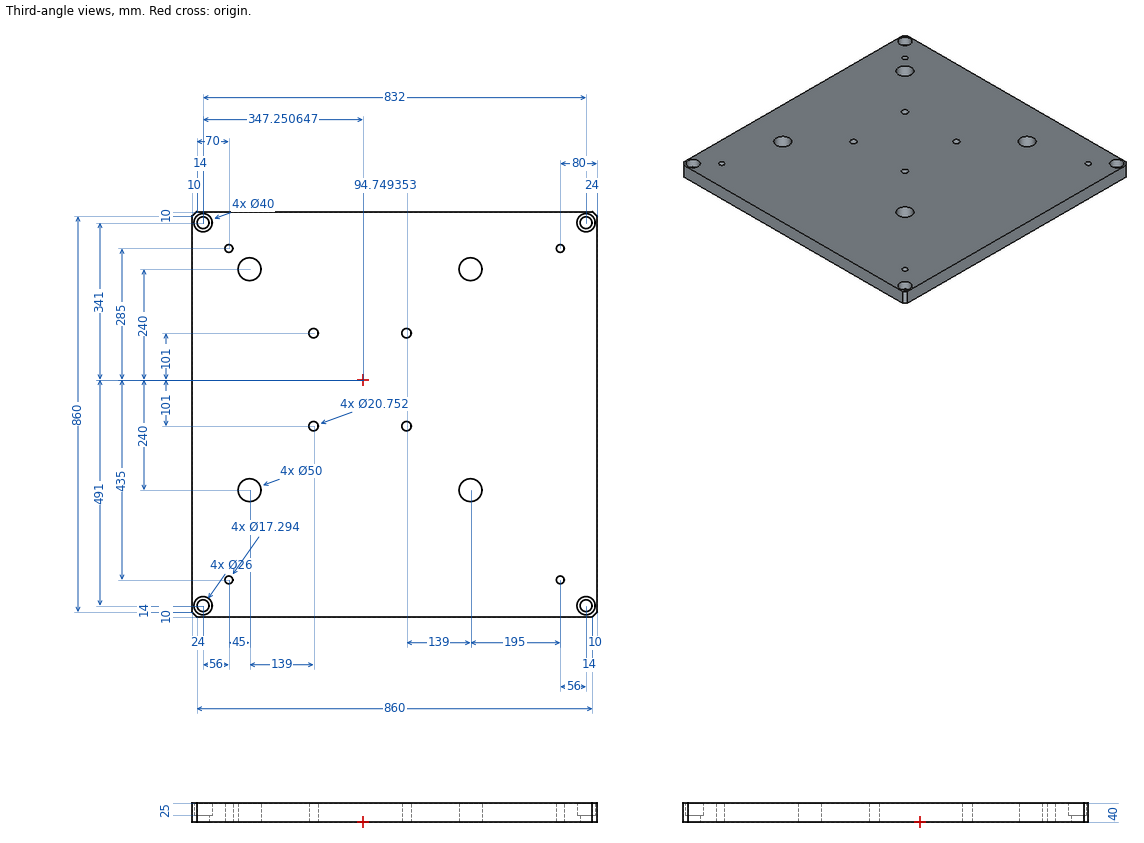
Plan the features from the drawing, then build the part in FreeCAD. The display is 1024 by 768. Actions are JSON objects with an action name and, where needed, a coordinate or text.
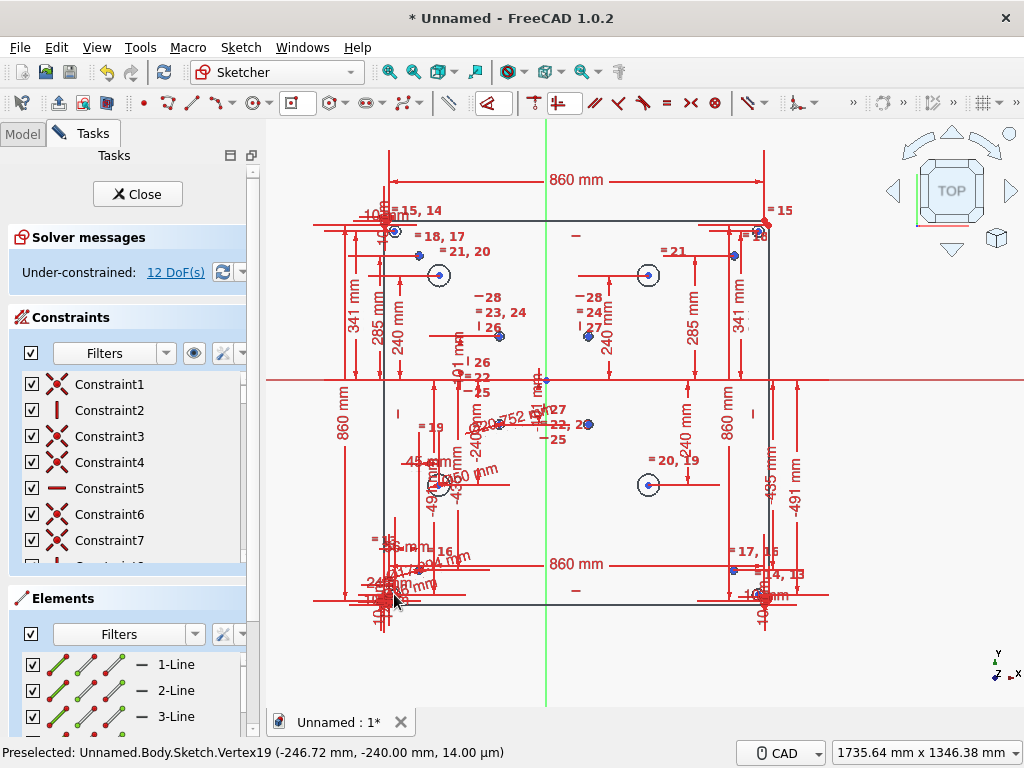
{"action": "scroll", "coordinate": [764, 605], "scroll_direction": "up", "scroll_amount": 10}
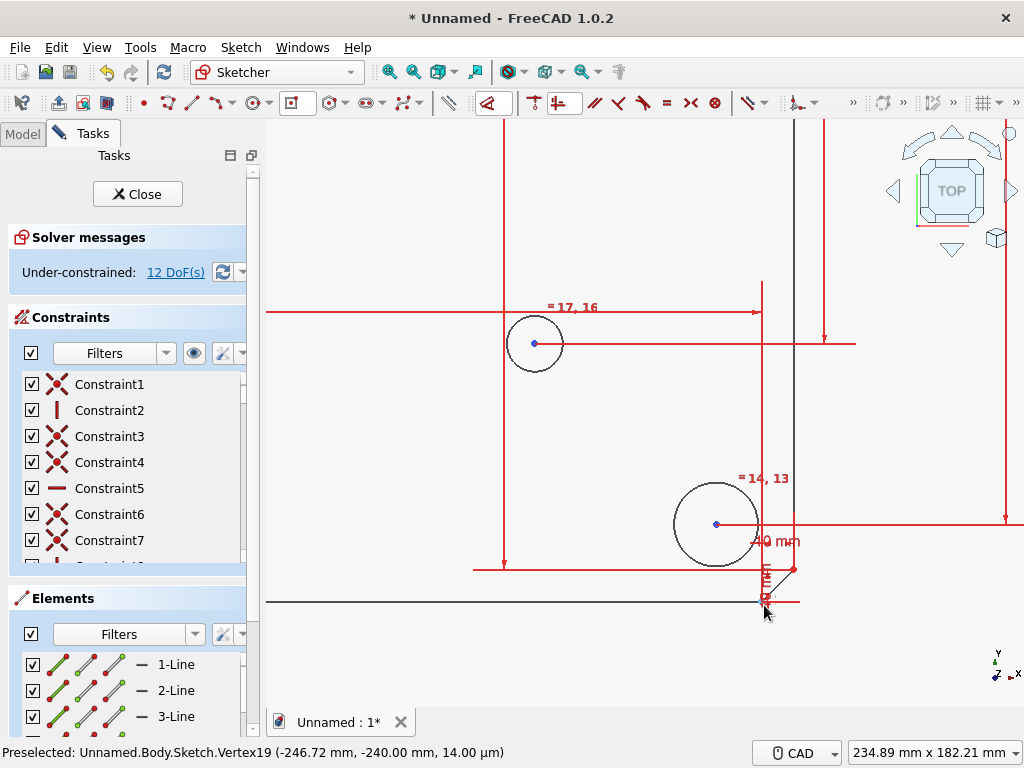
{"action": "left_click", "coordinate": [762, 602]}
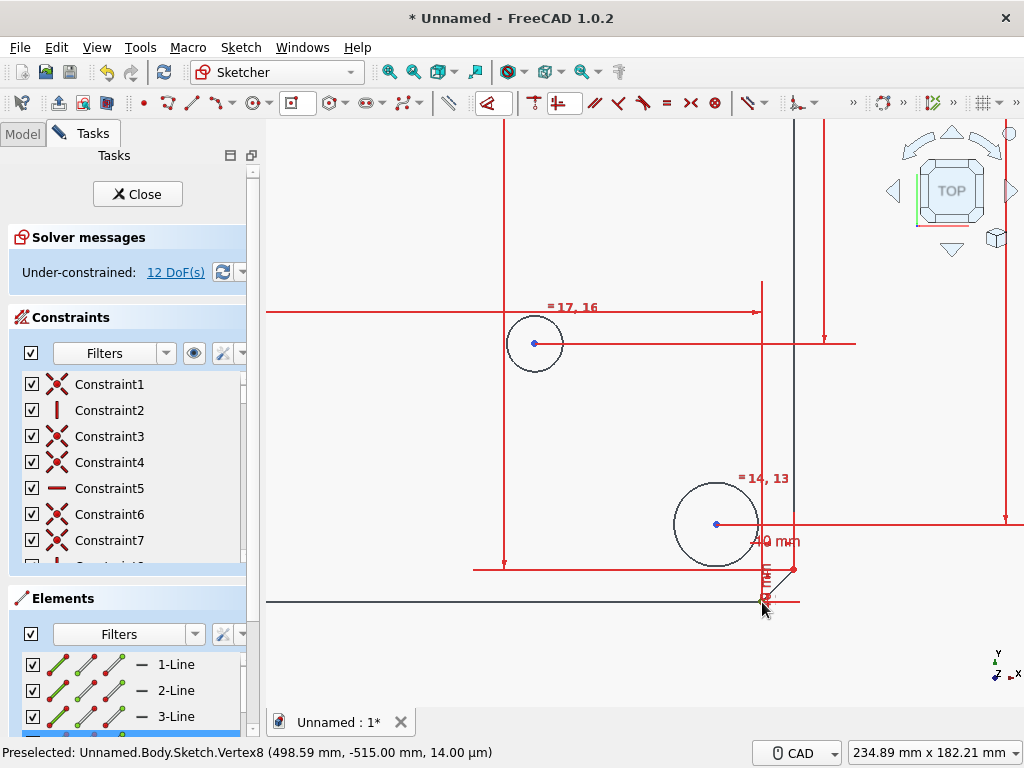
{"action": "left_click", "coordinate": [716, 525]}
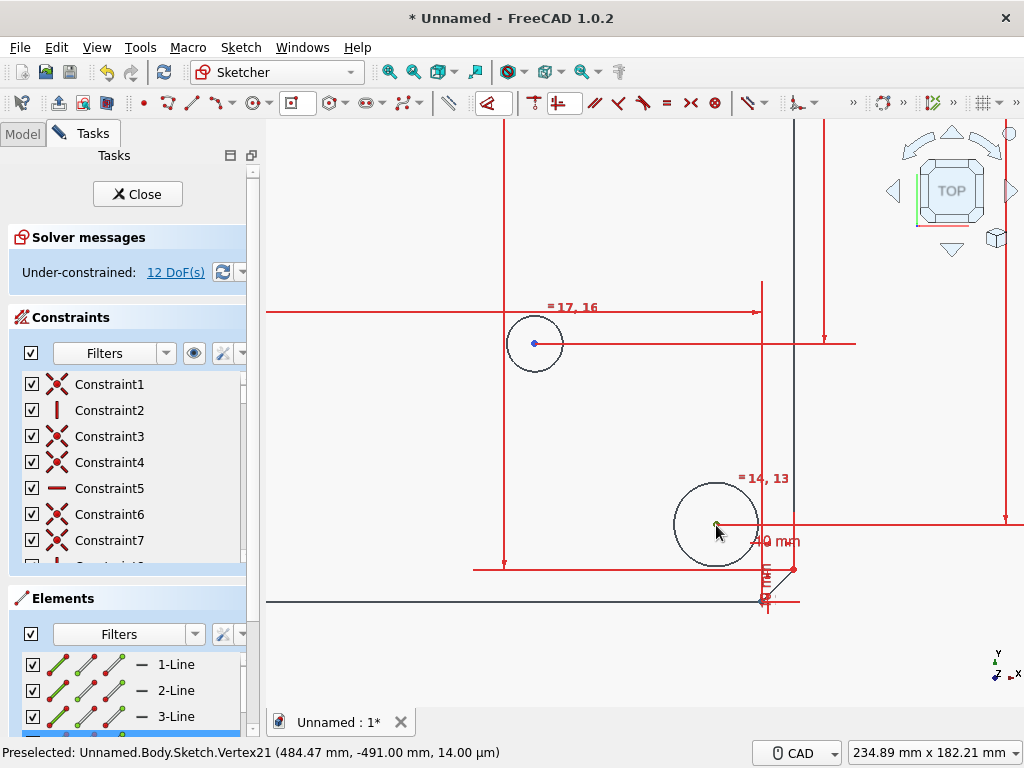
{"action": "key", "text": "l"}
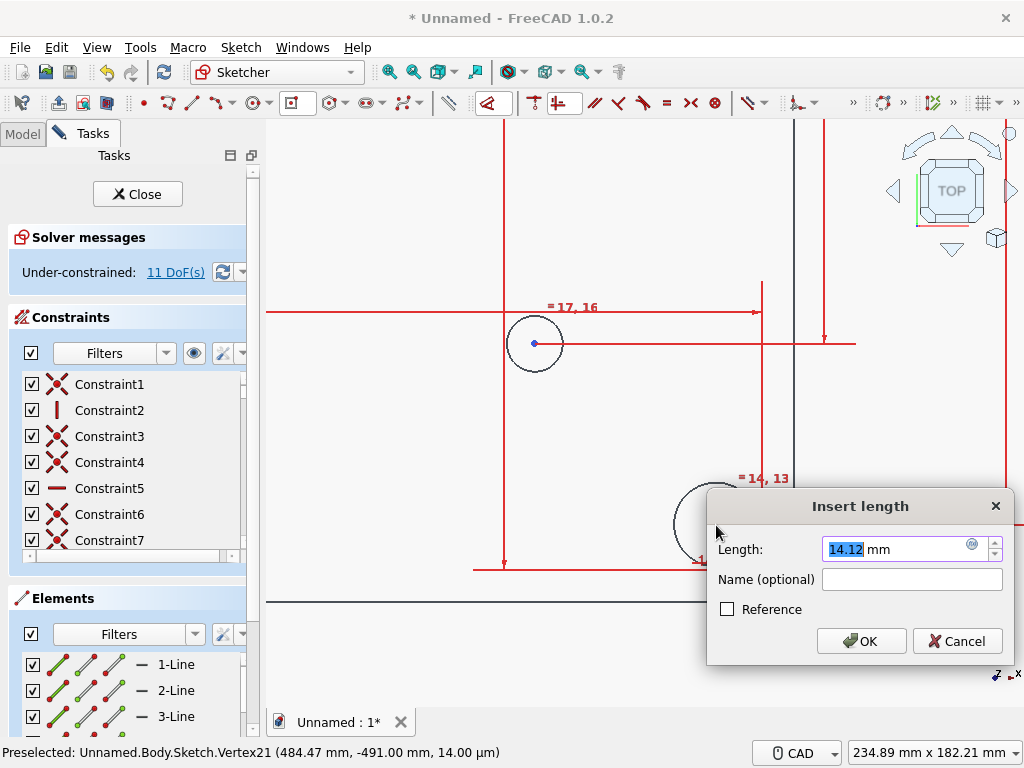
{"action": "type", "text": "14"}
{"action": "key", "text": "Return"}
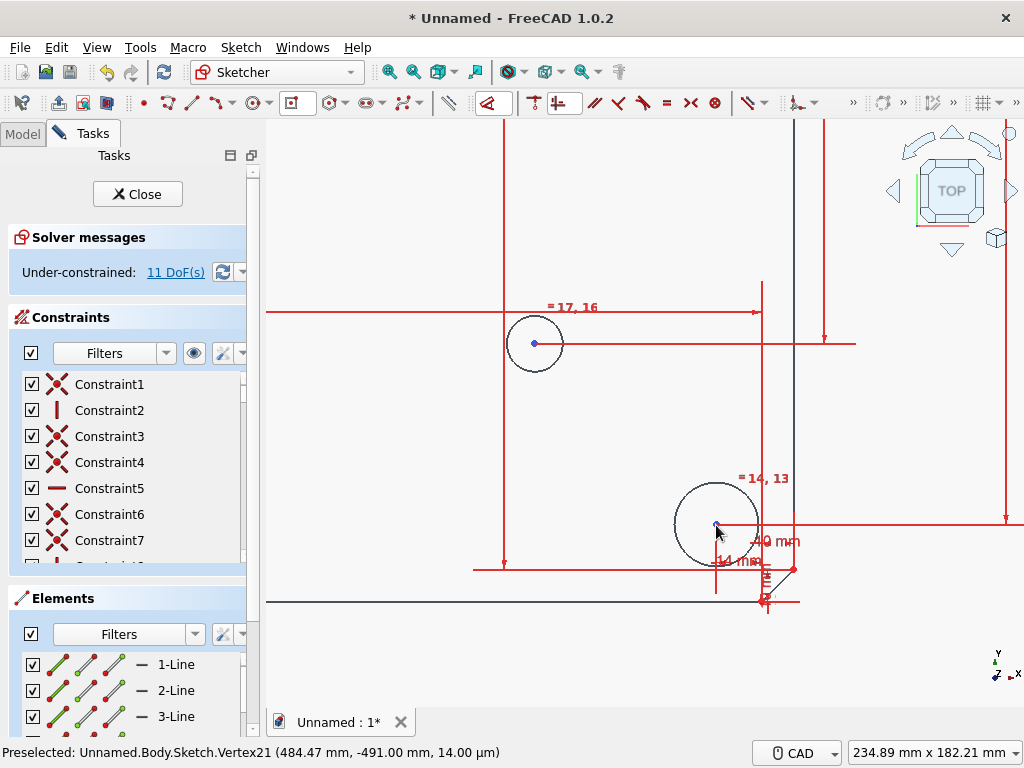
{"action": "scroll", "coordinate": [765, 606], "scroll_direction": "down", "scroll_amount": 10}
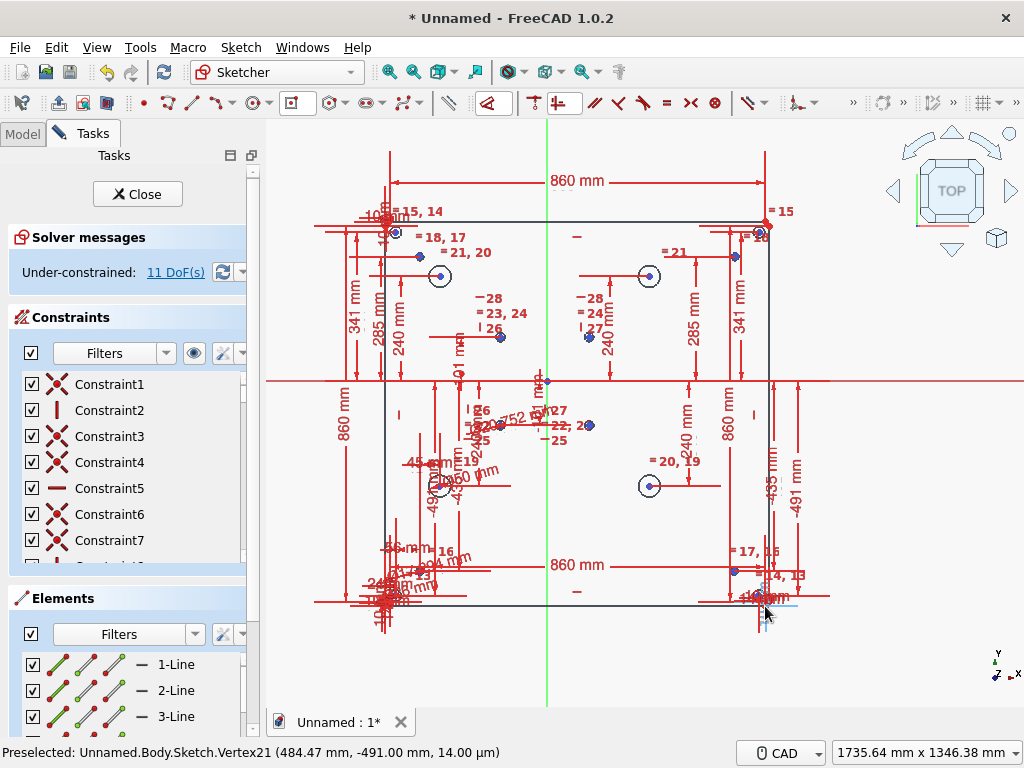
{"action": "scroll", "coordinate": [759, 596], "scroll_direction": "up", "scroll_amount": 3}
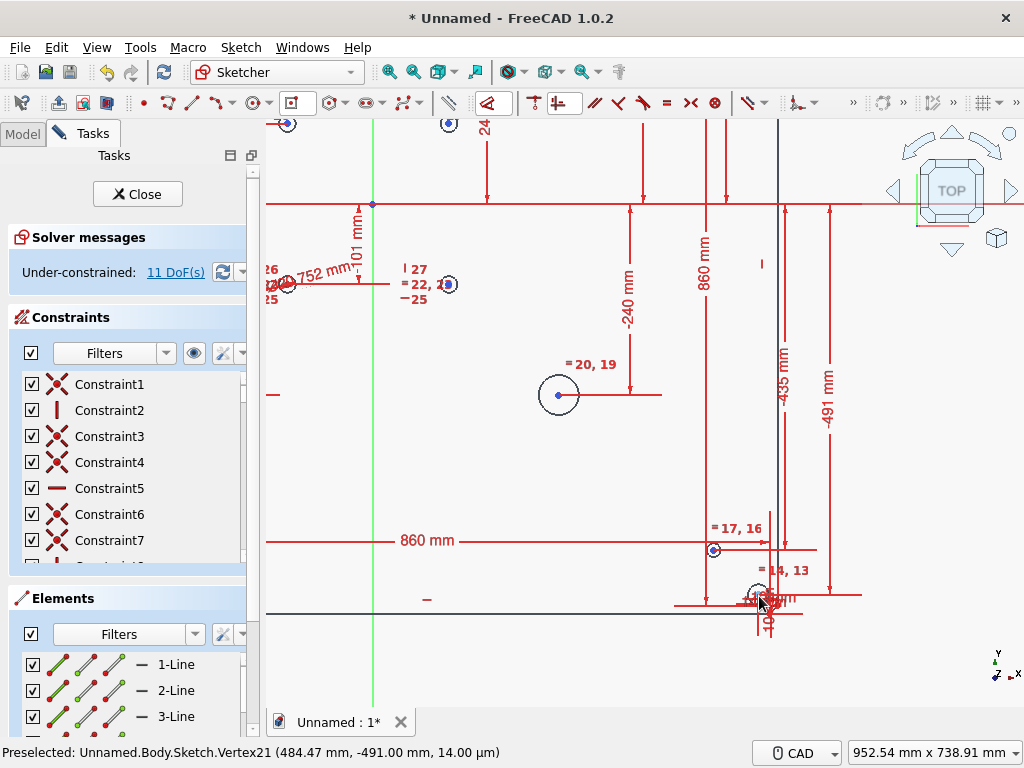
{"action": "left_click", "coordinate": [758, 595]}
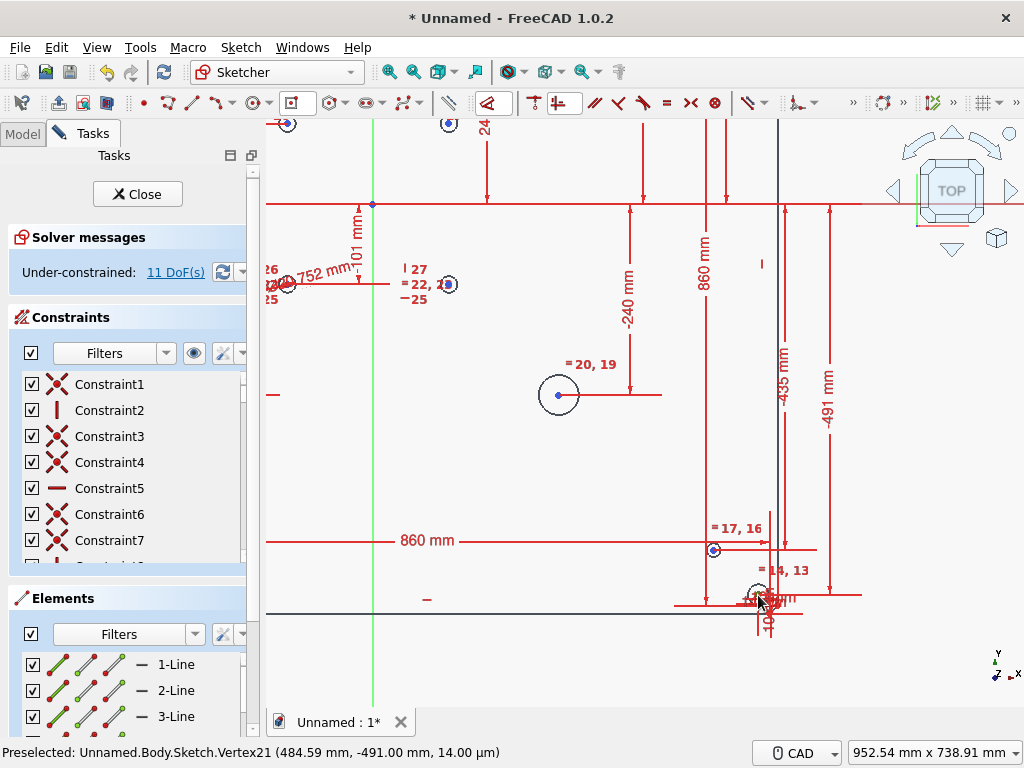
{"action": "left_click", "coordinate": [714, 550]}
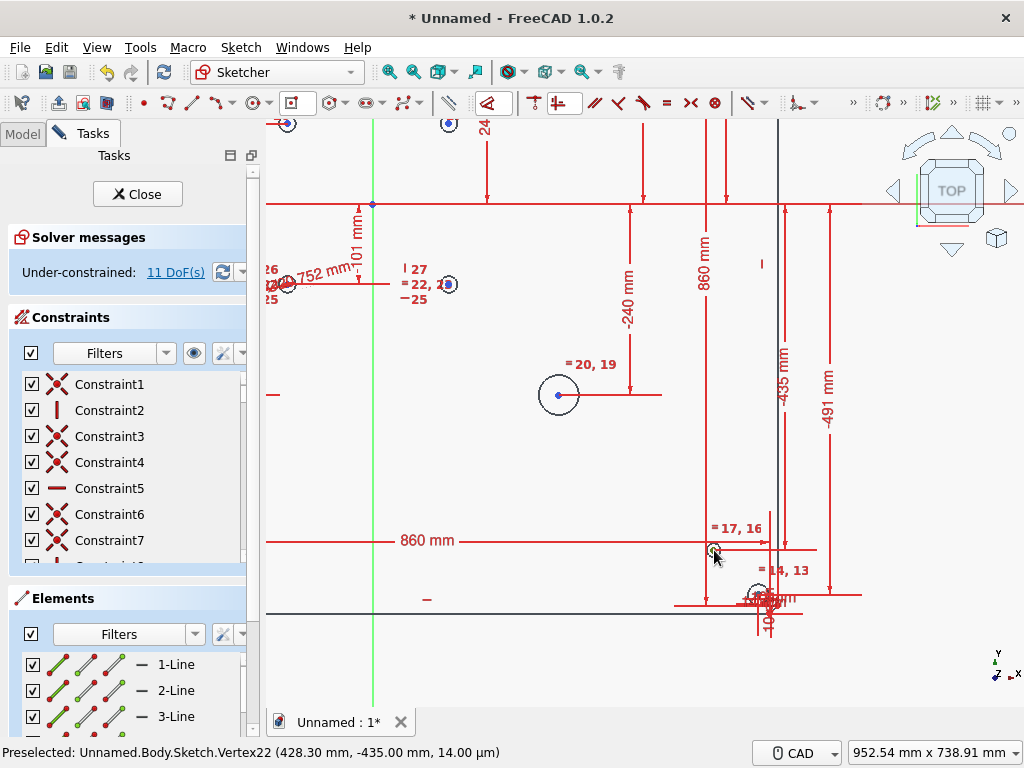
{"action": "key", "text": "l"}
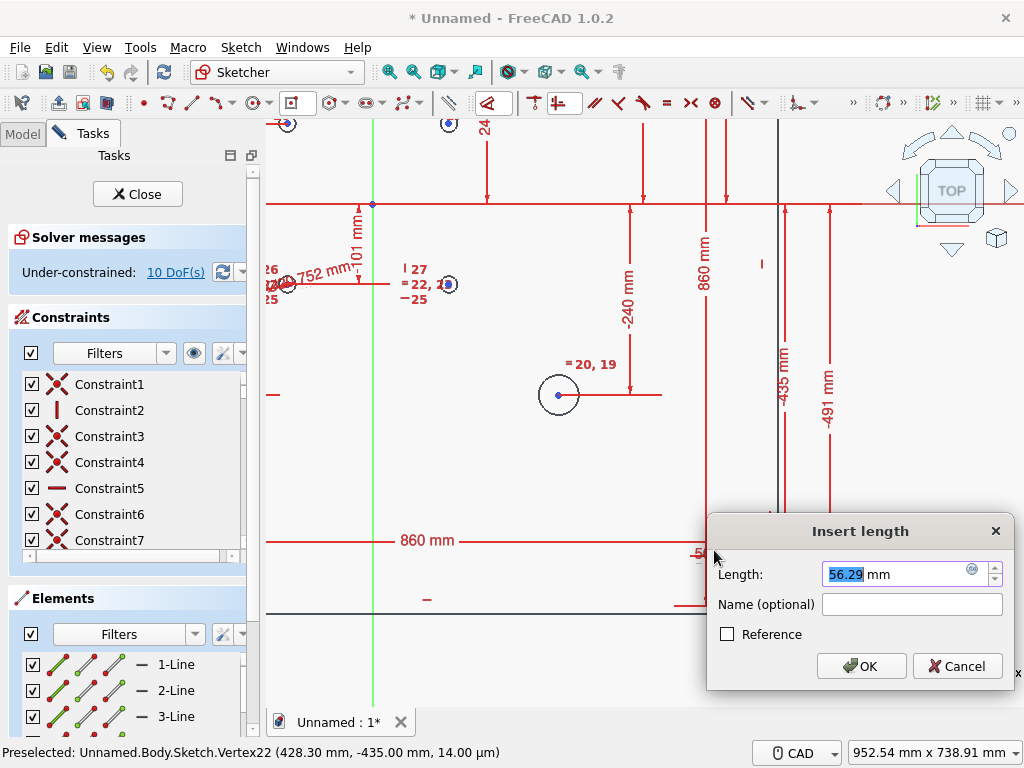
{"action": "type", "text": "56"}
{"action": "key", "text": "Return"}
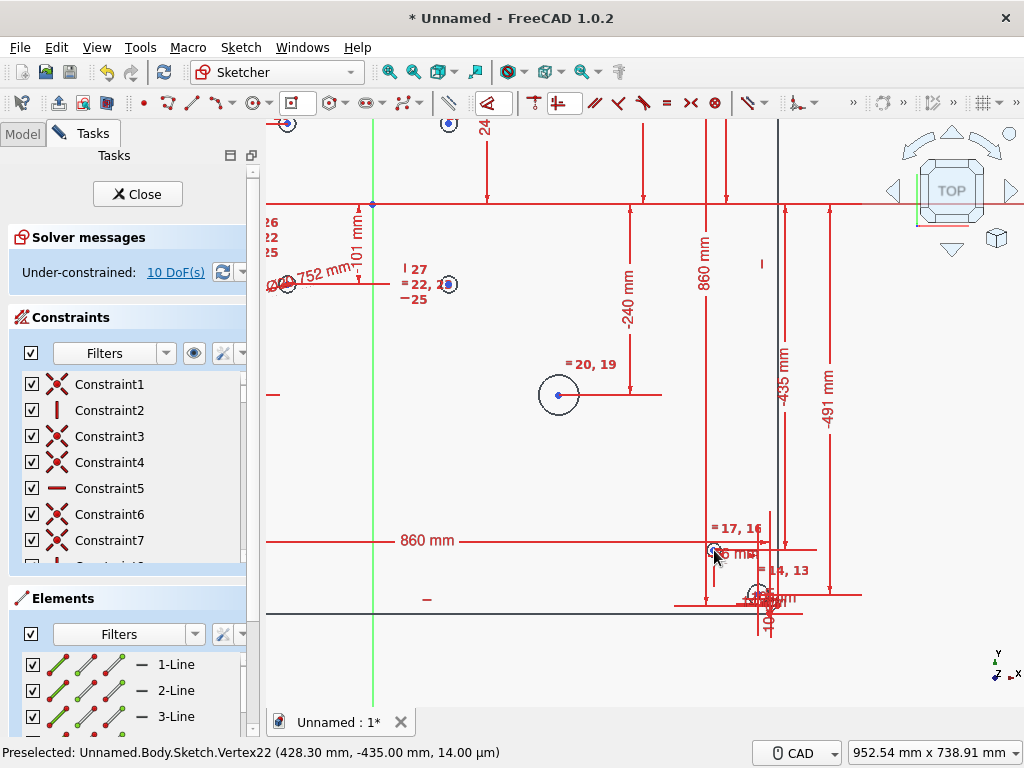
{"action": "scroll", "coordinate": [758, 595], "scroll_direction": "down", "scroll_amount": 3}